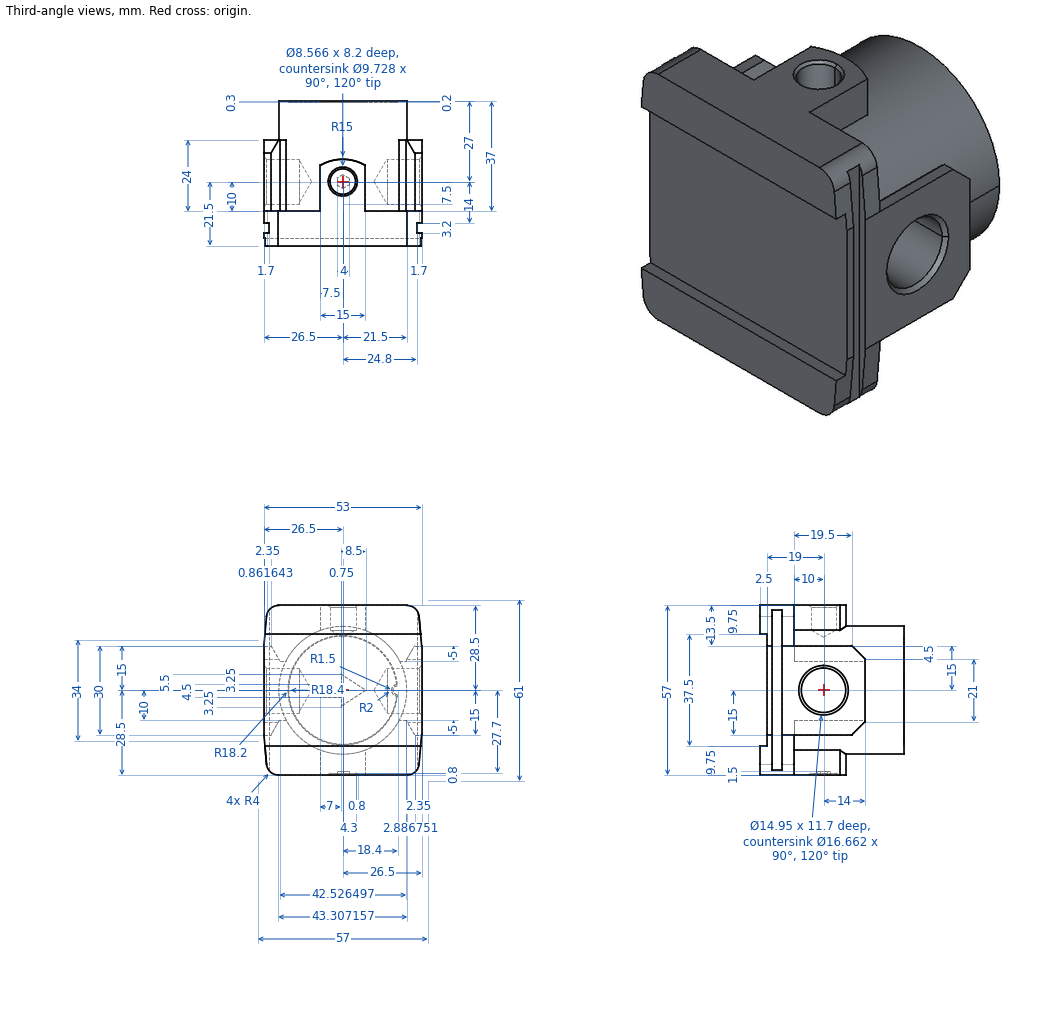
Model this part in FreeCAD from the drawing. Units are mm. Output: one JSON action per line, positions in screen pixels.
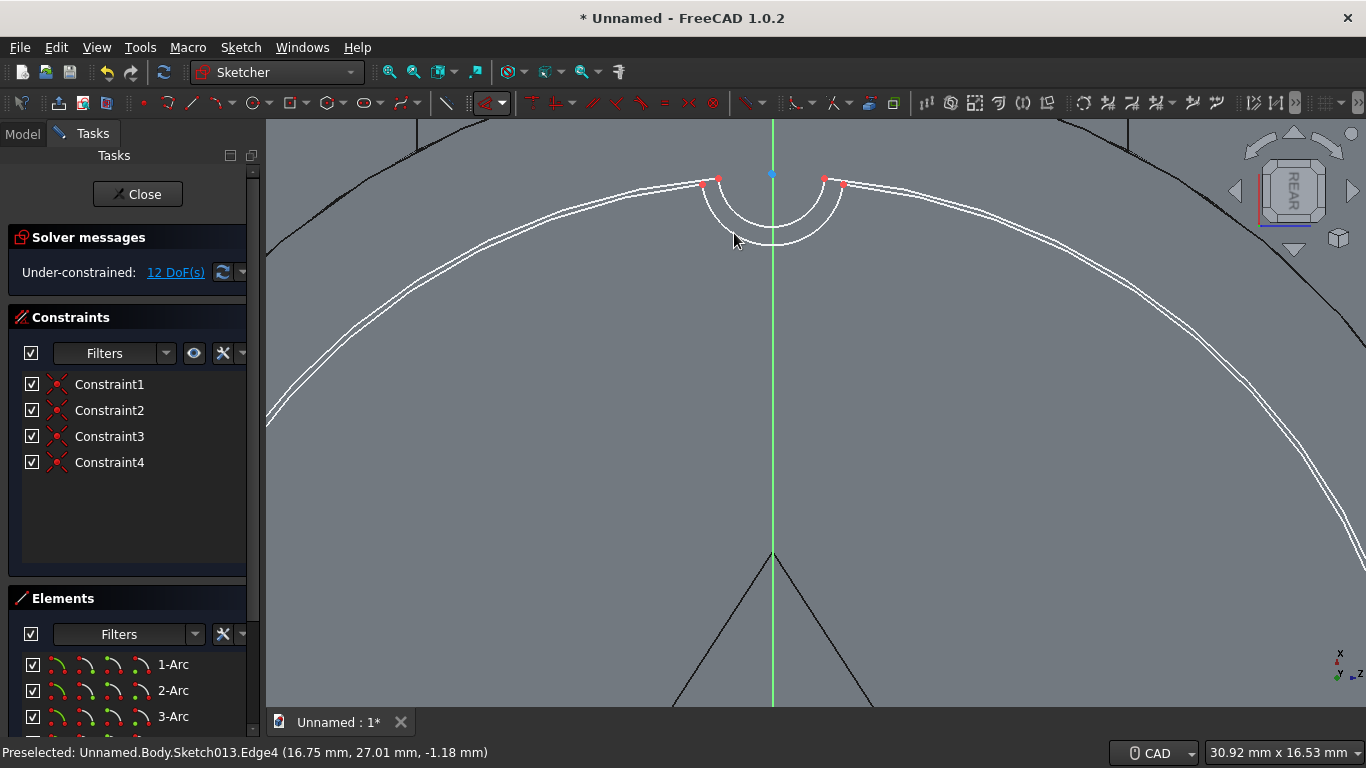
{"action": "scroll", "coordinate": [737, 234], "scroll_direction": "down", "scroll_amount": 6}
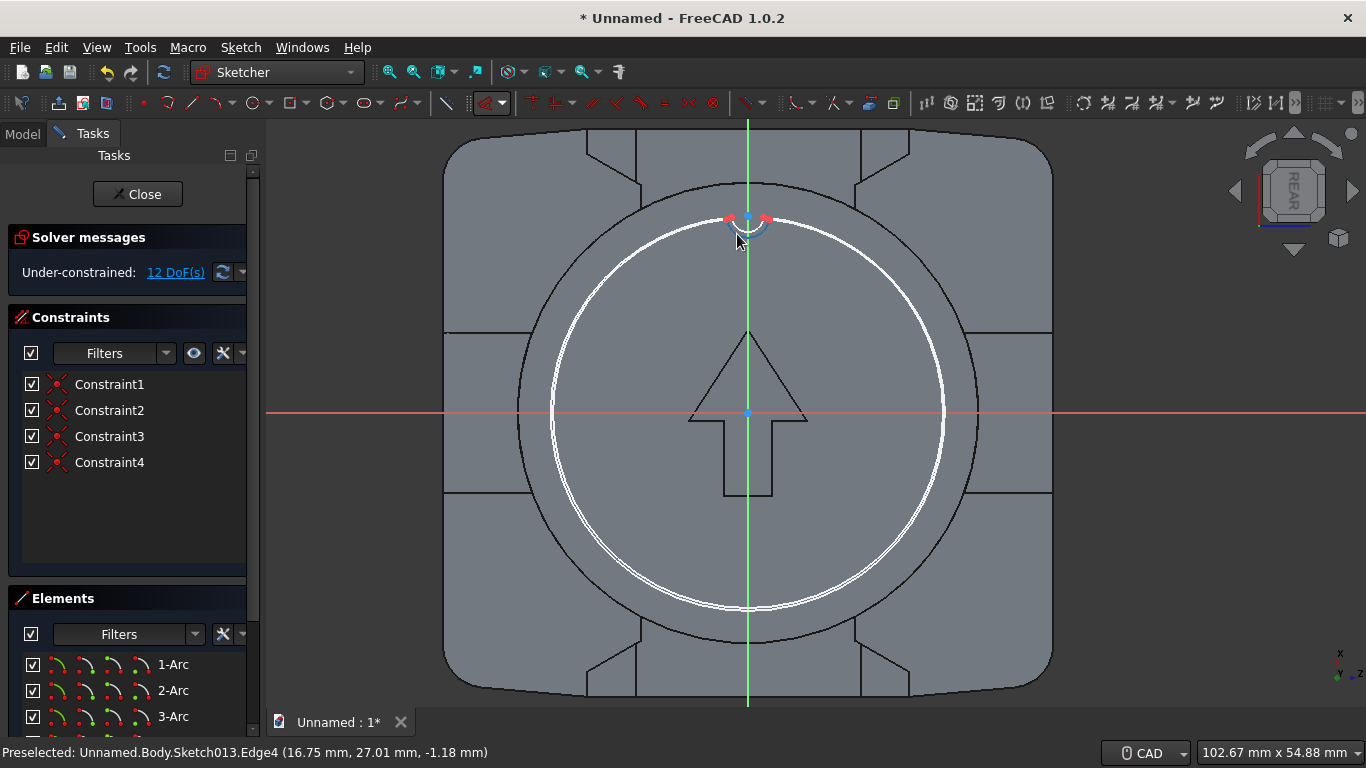
{"action": "scroll", "coordinate": [748, 611], "scroll_direction": "up", "scroll_amount": 8}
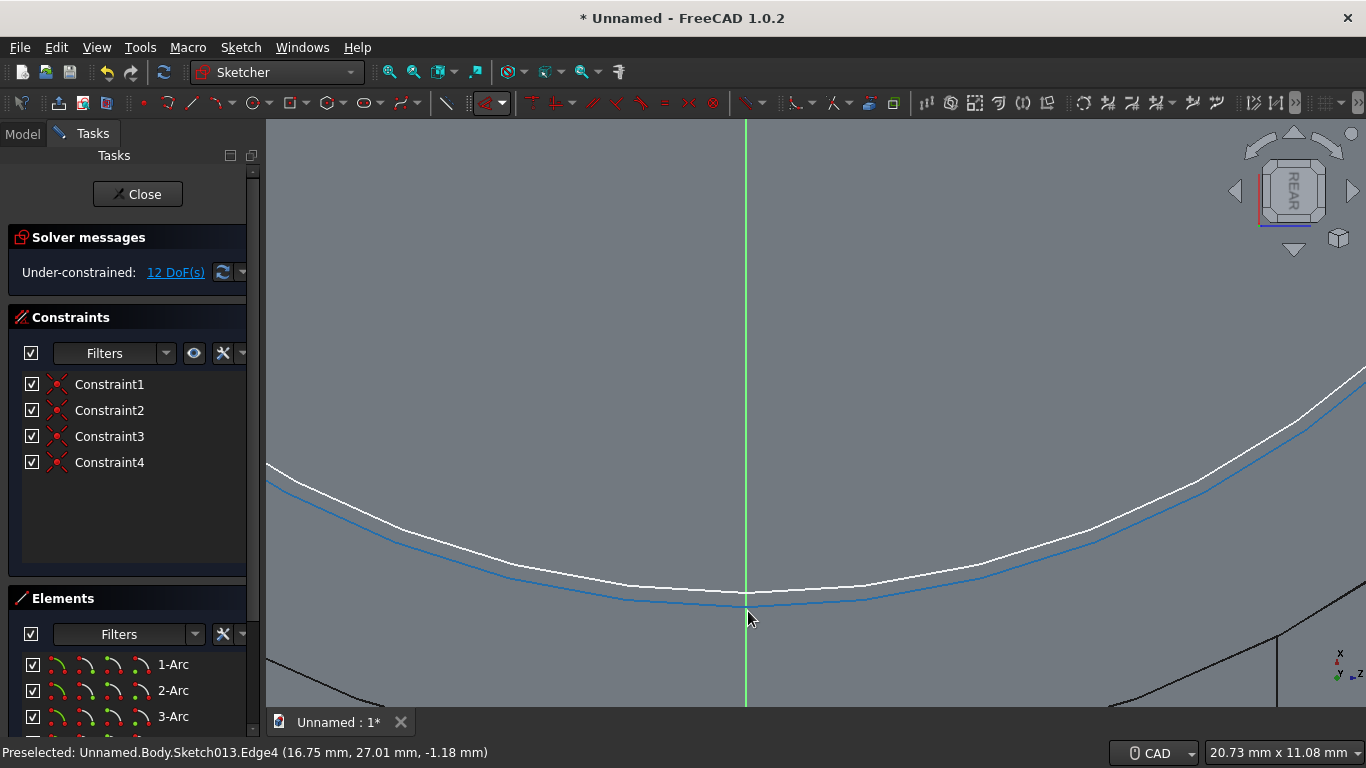
{"action": "left_click", "coordinate": [745, 607]}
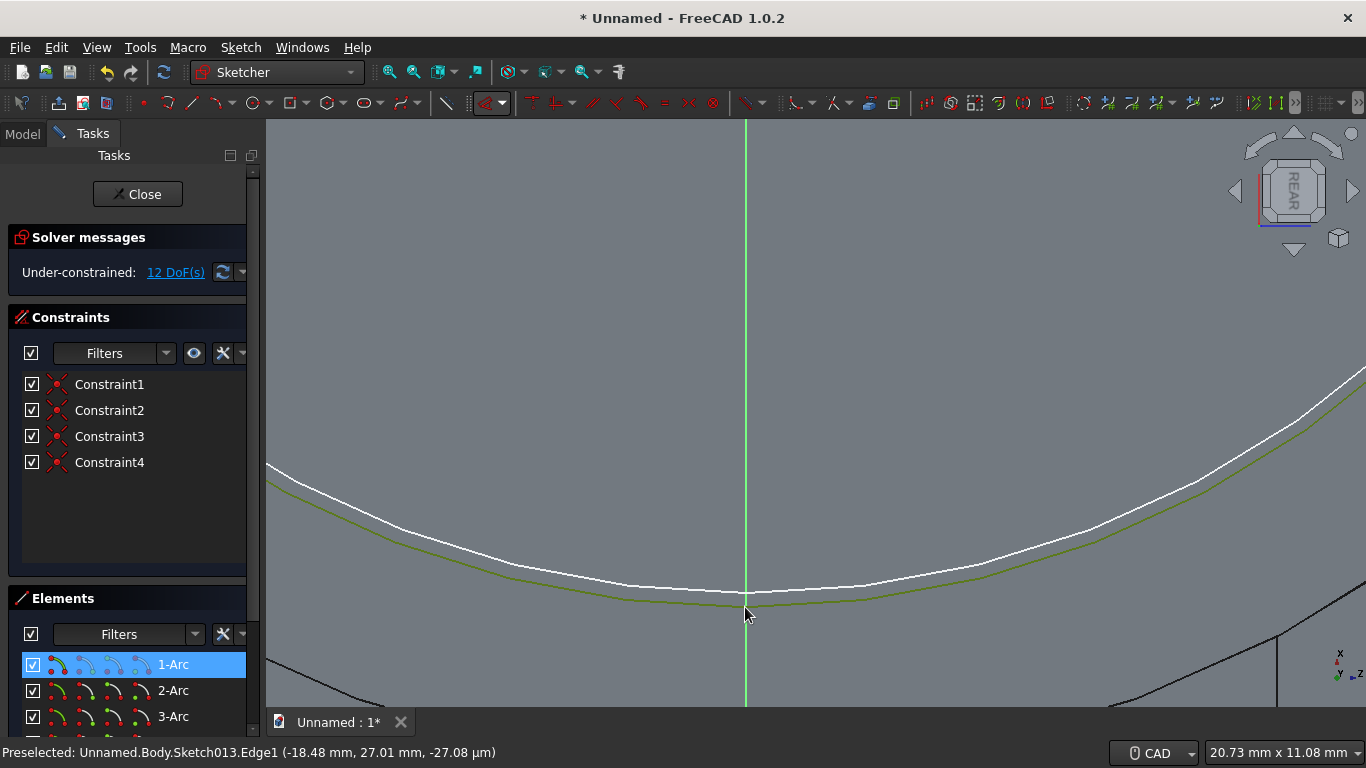
{"action": "left_click", "coordinate": [746, 593]}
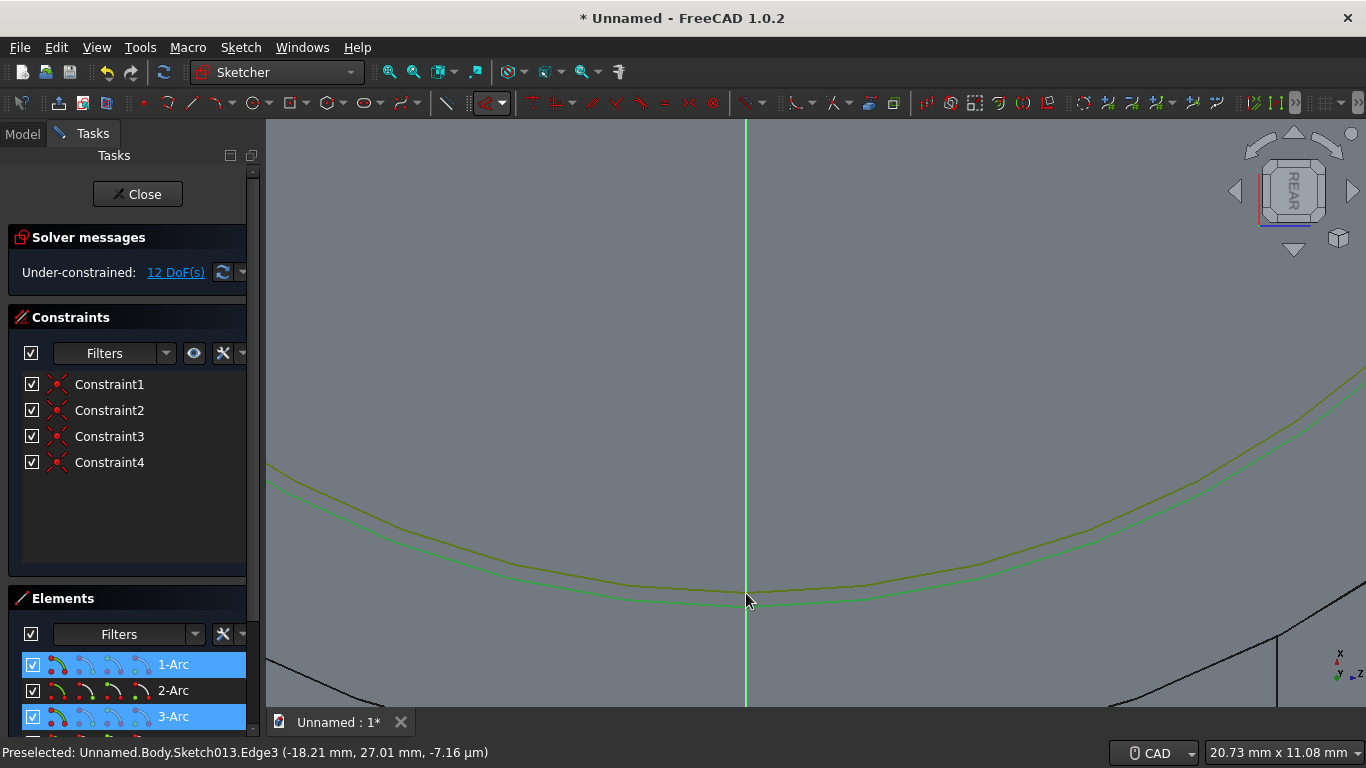
{"action": "key", "text": "c"}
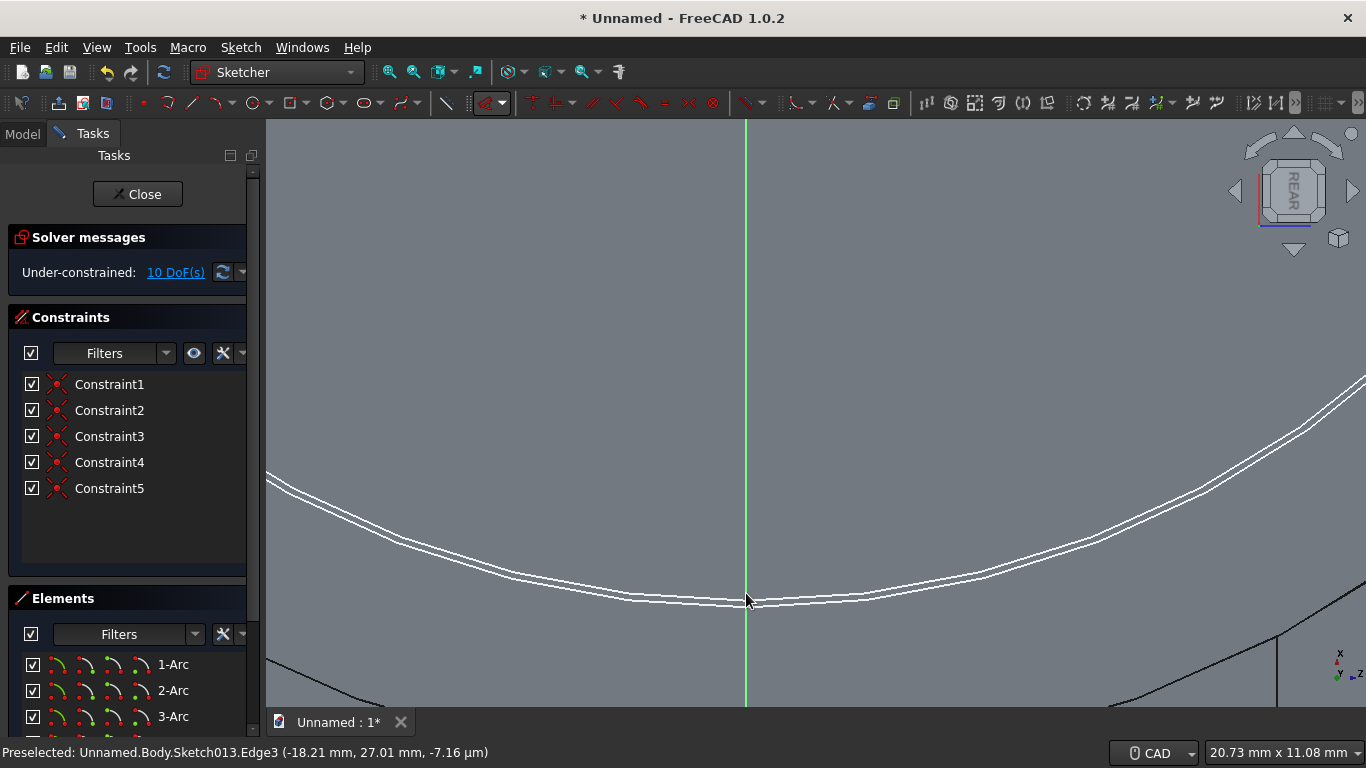
{"action": "scroll", "coordinate": [748, 612], "scroll_direction": "down", "scroll_amount": 8}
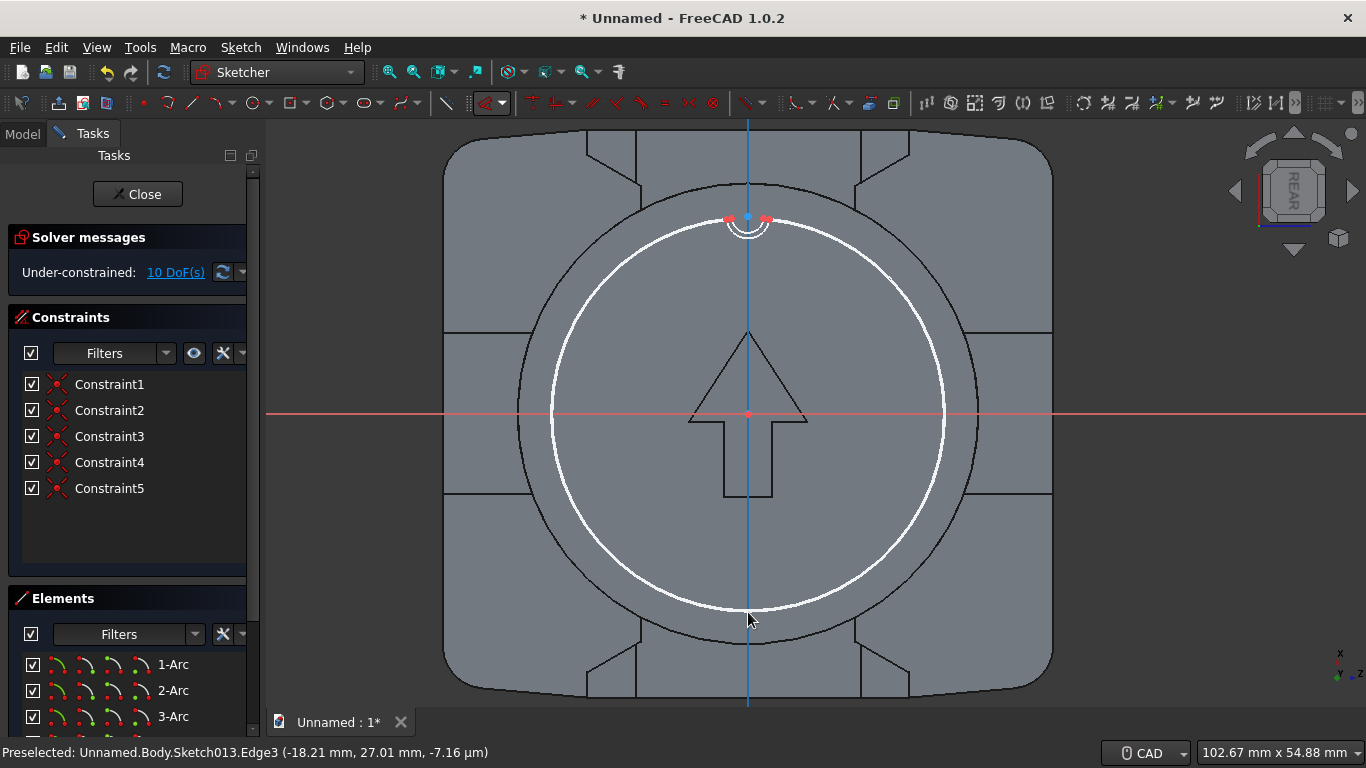
{"action": "scroll", "coordinate": [739, 230], "scroll_direction": "up", "scroll_amount": 5}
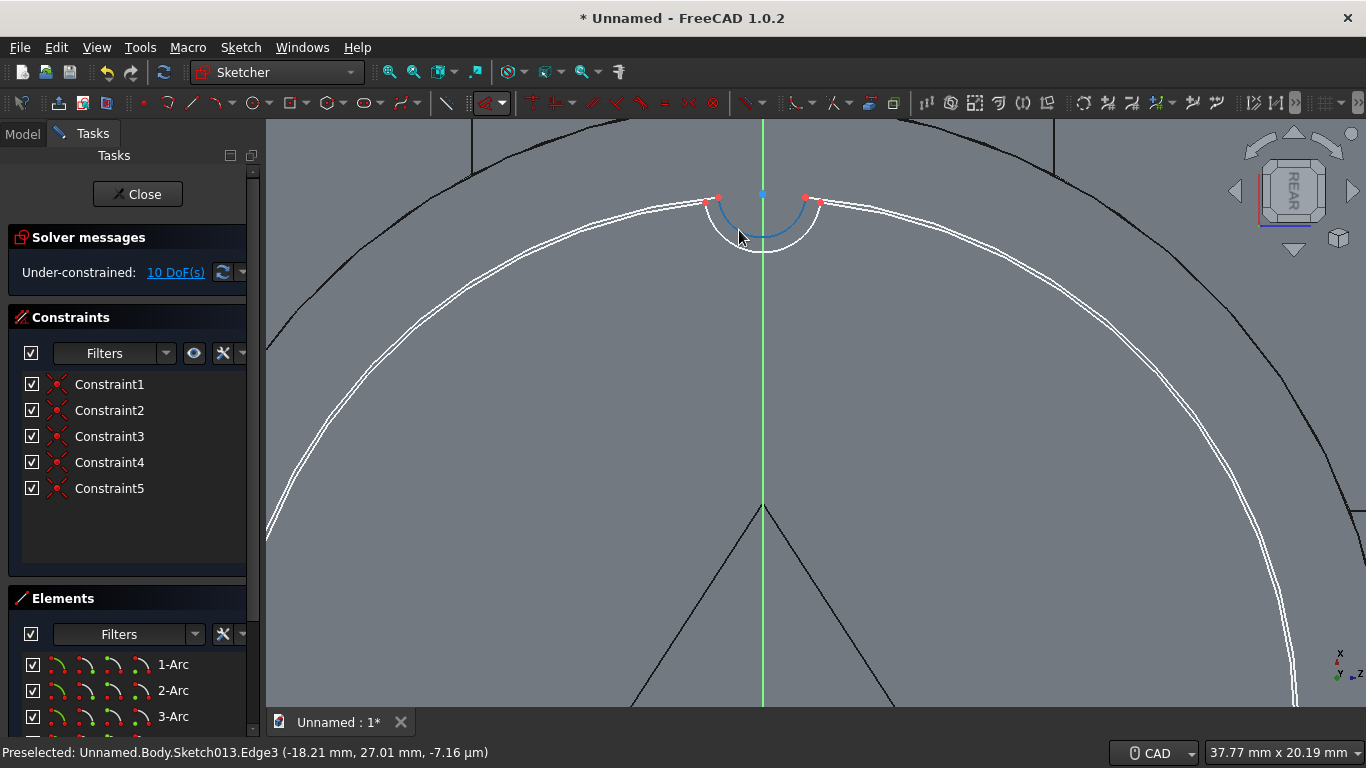
{"action": "left_click", "coordinate": [738, 230]}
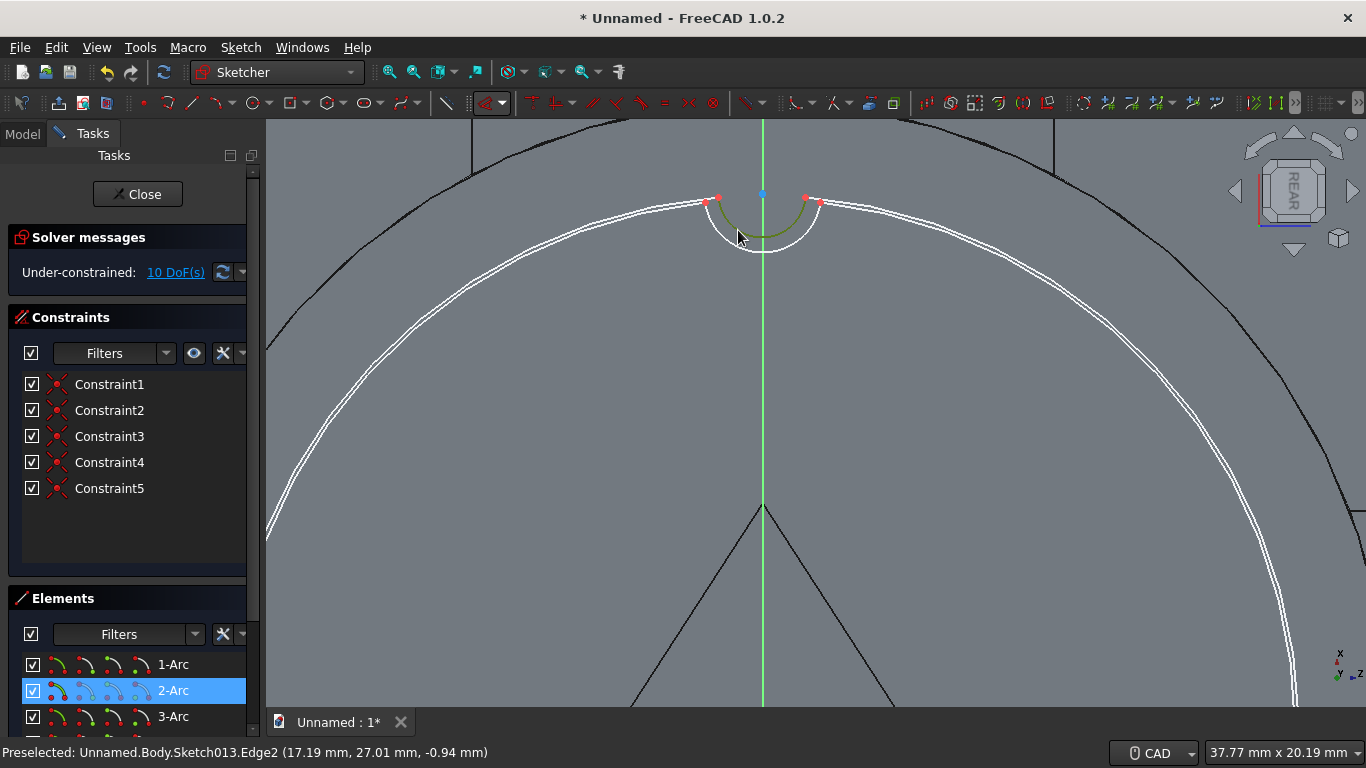
{"action": "left_click", "coordinate": [731, 243]}